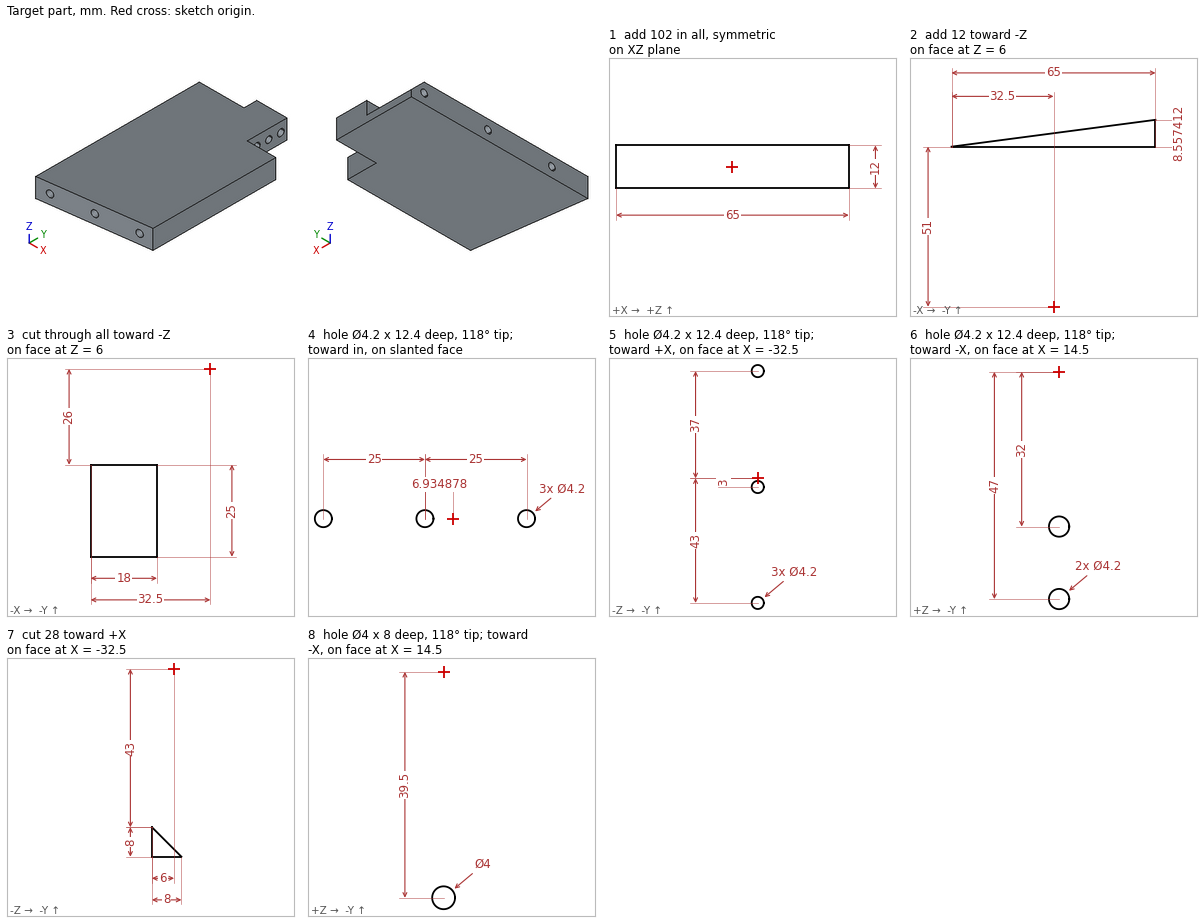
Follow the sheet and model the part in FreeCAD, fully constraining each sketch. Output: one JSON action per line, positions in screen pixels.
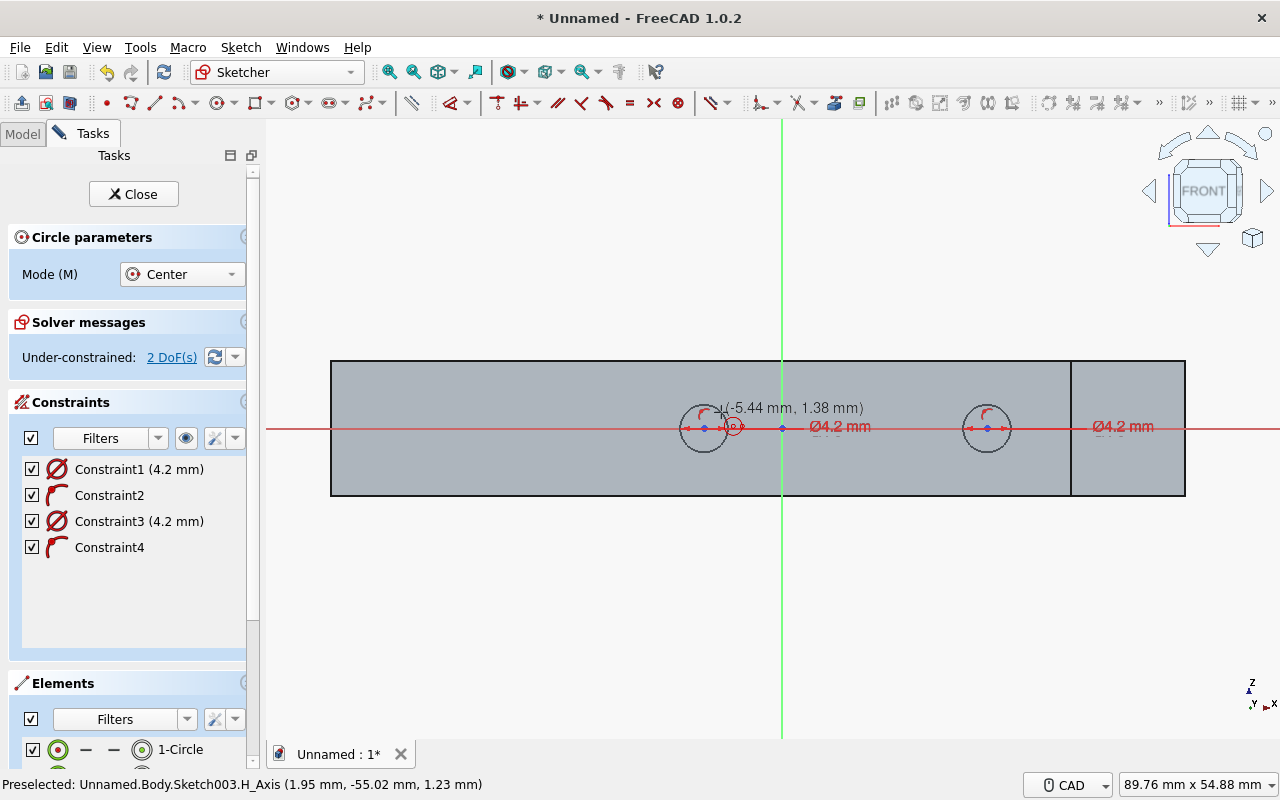
{"action": "left_click", "coordinate": [422, 429]}
{"action": "mouse_move", "coordinate": [438, 412]}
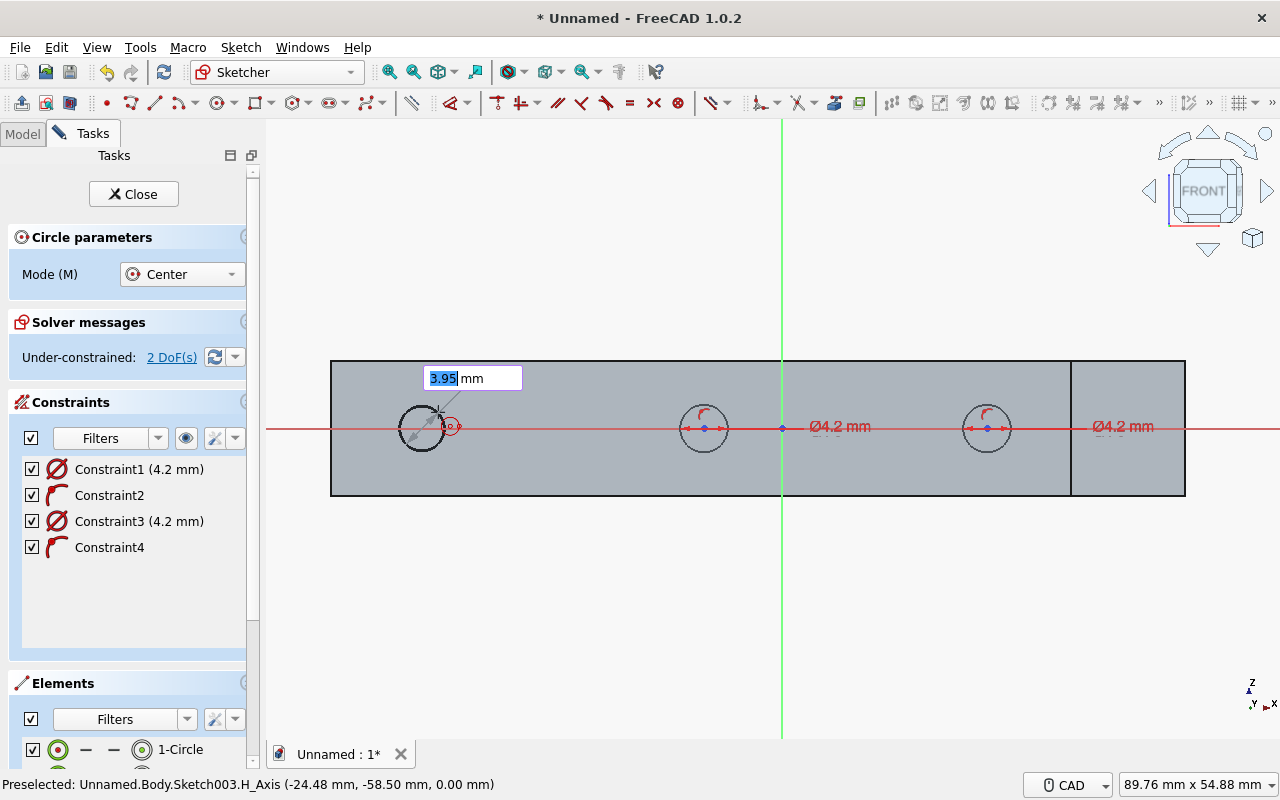
{"action": "type", "text": "4.2"}
{"action": "key", "text": "Return"}
{"action": "key", "text": "Escape"}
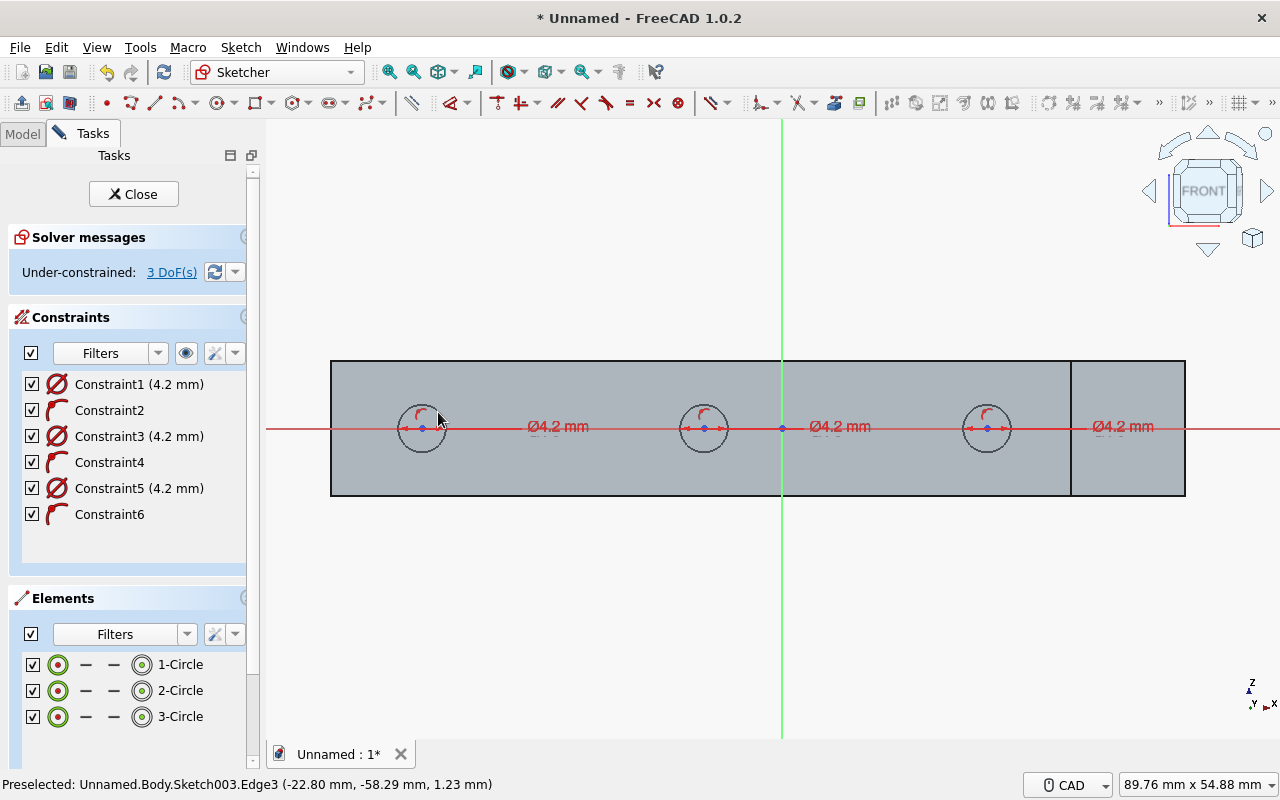
{"action": "key", "text": "d"}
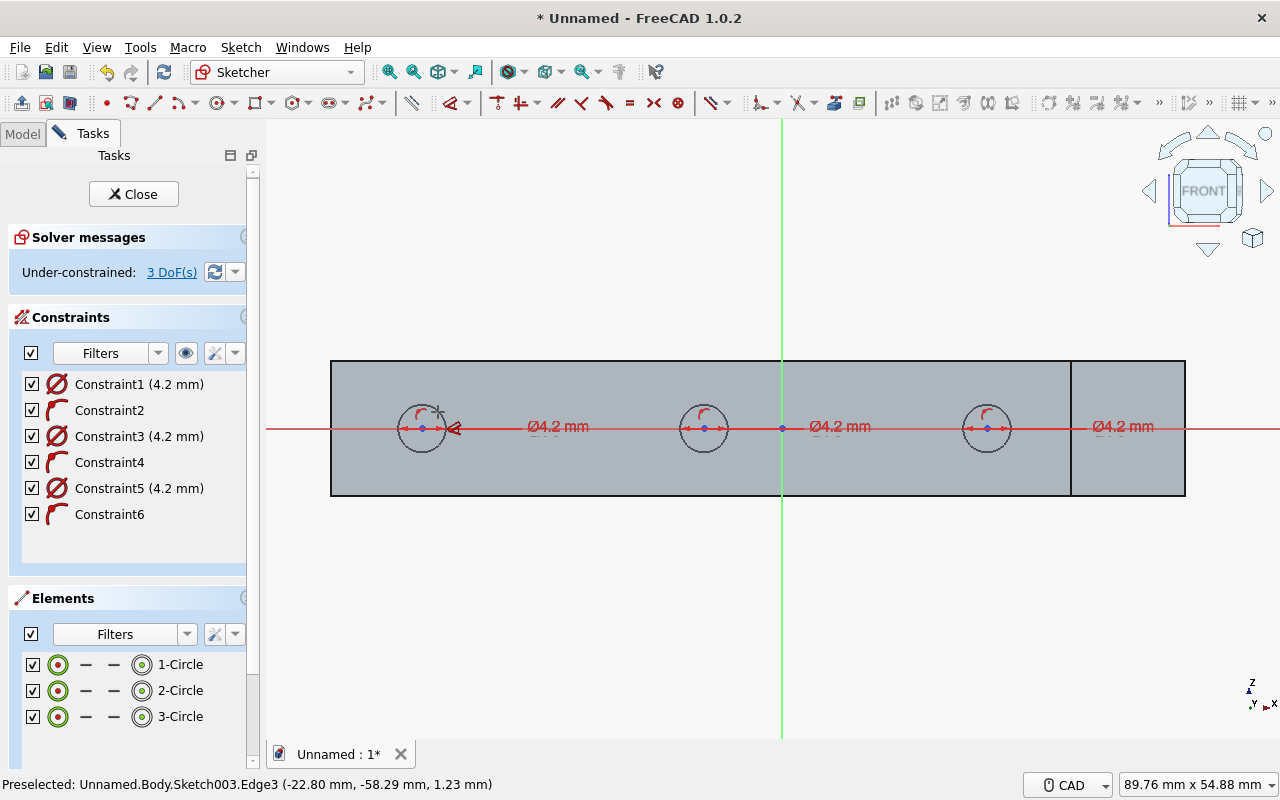
{"action": "left_click", "coordinate": [987, 429]}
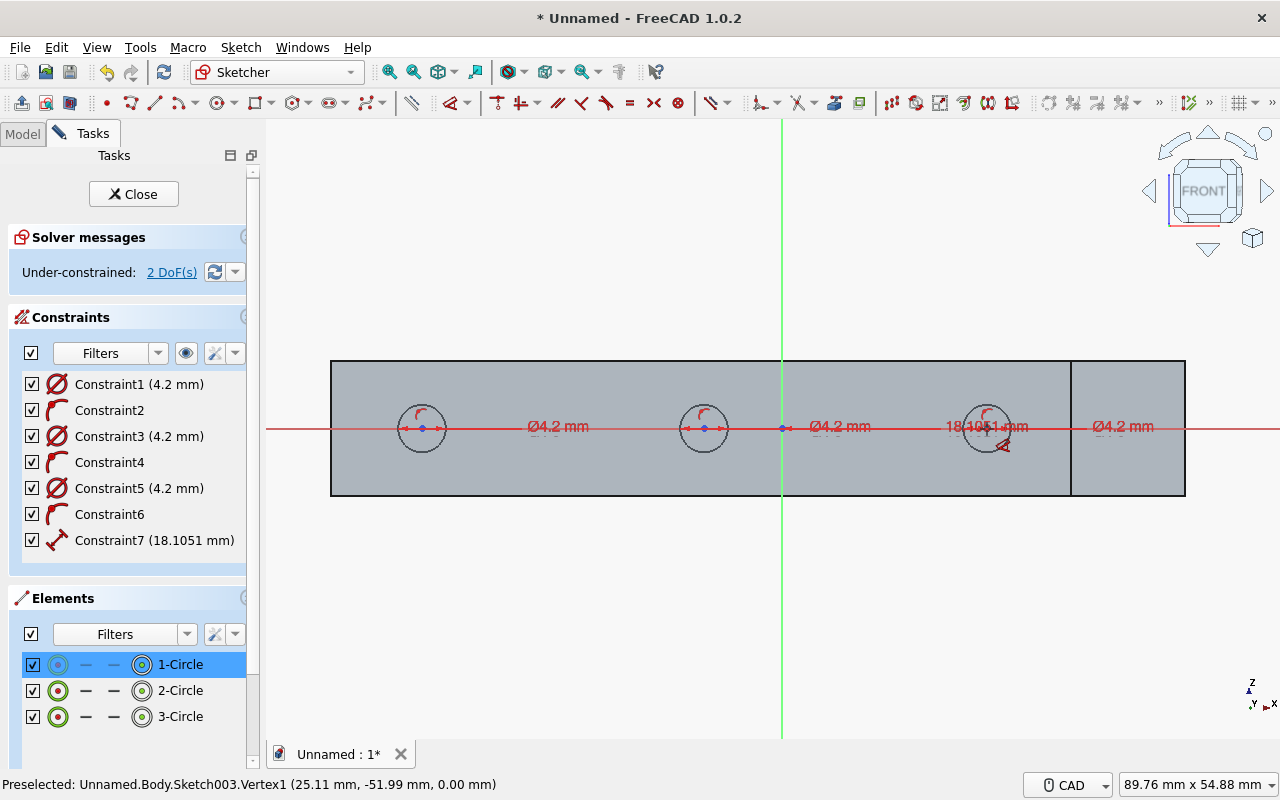
{"action": "left_click", "coordinate": [704, 429]}
{"action": "left_click", "coordinate": [845, 463]}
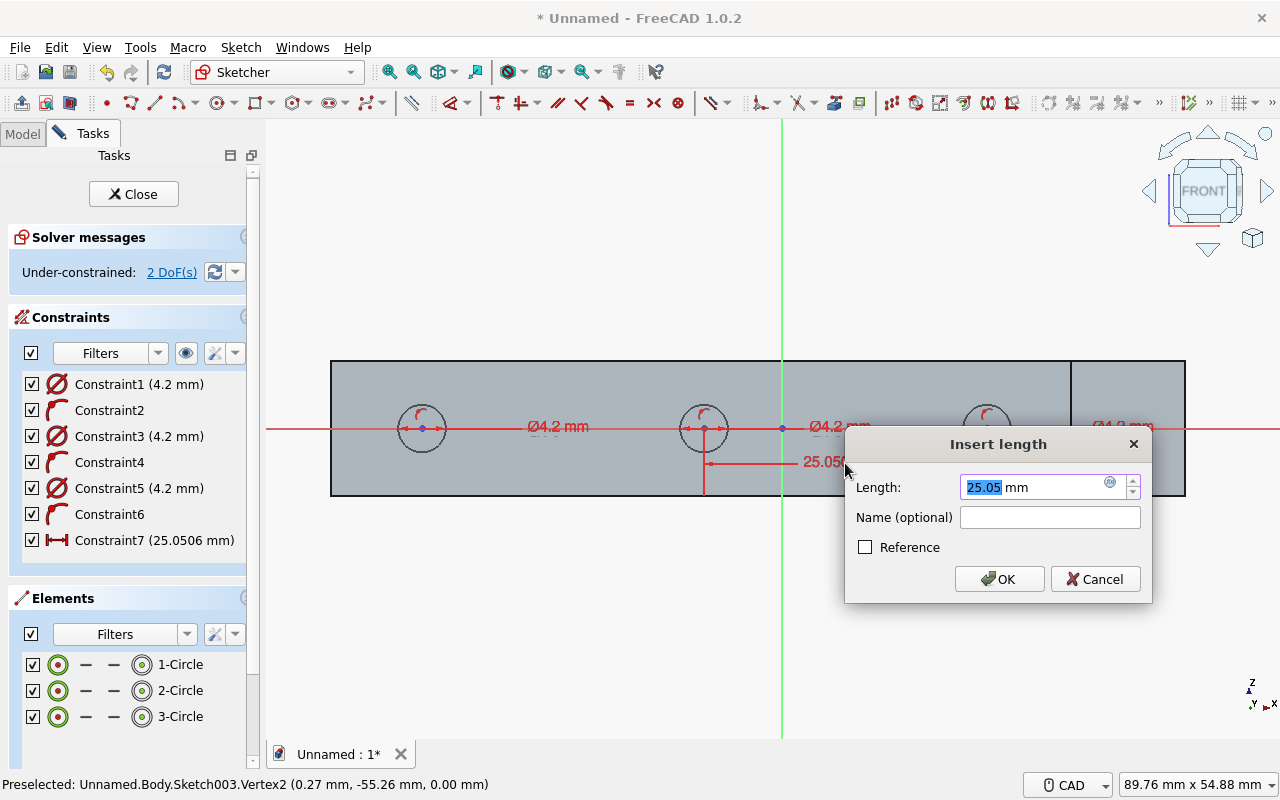
{"action": "type", "text": "25"}
{"action": "key", "text": "Return"}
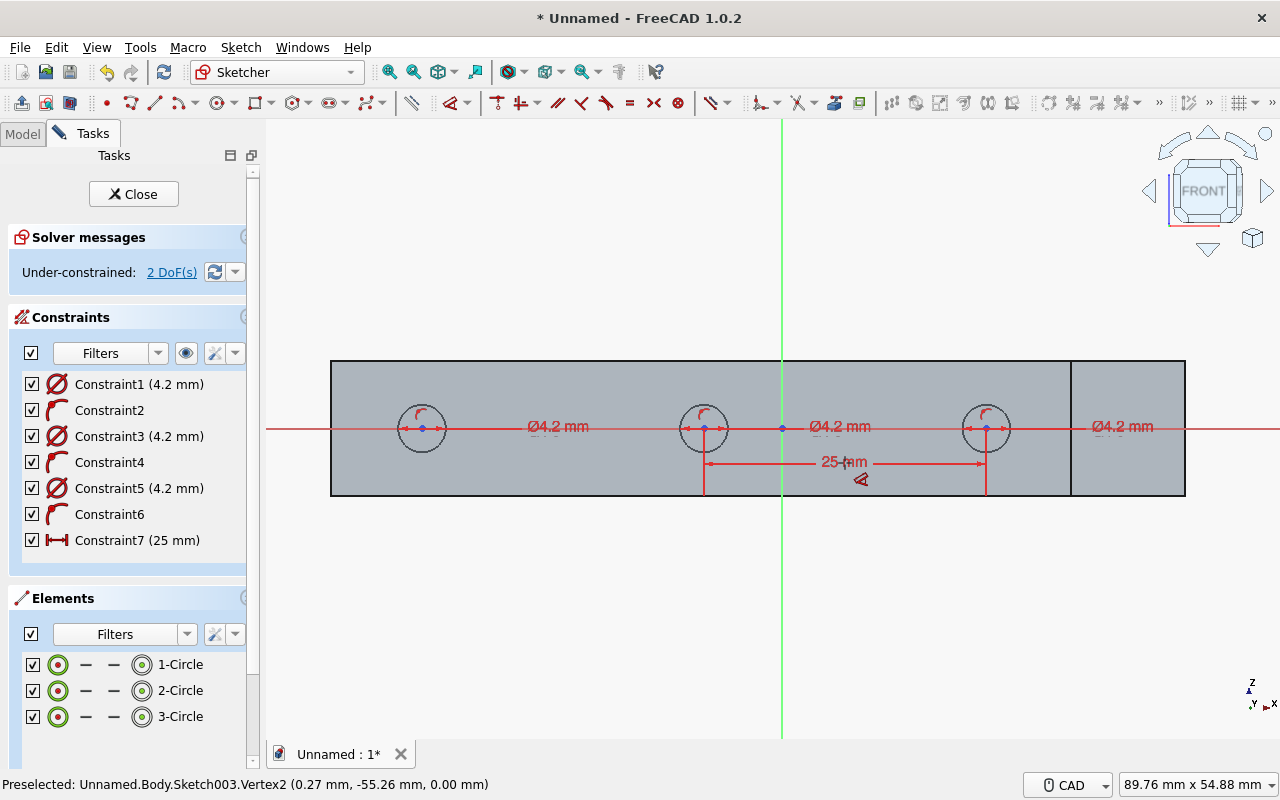
{"action": "left_click", "coordinate": [704, 429]}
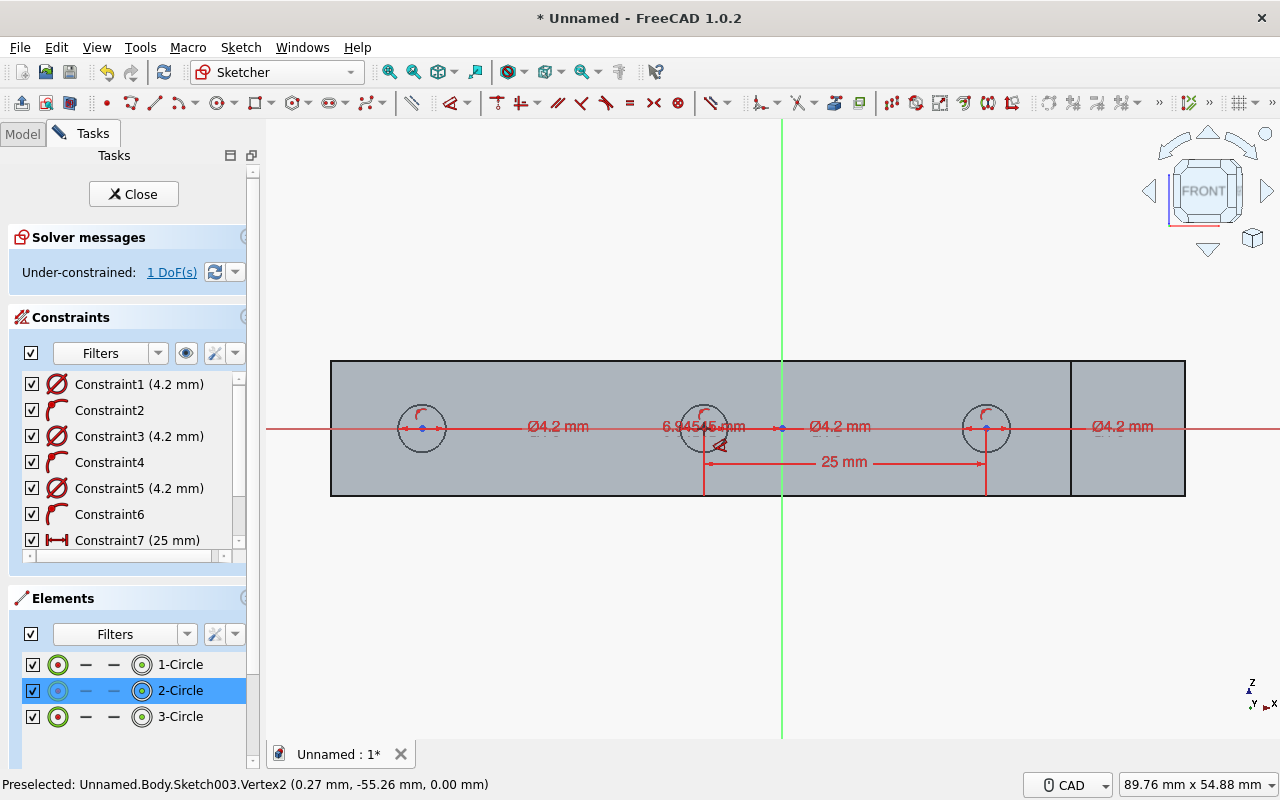
{"action": "left_click", "coordinate": [422, 429]}
{"action": "left_click", "coordinate": [563, 463]}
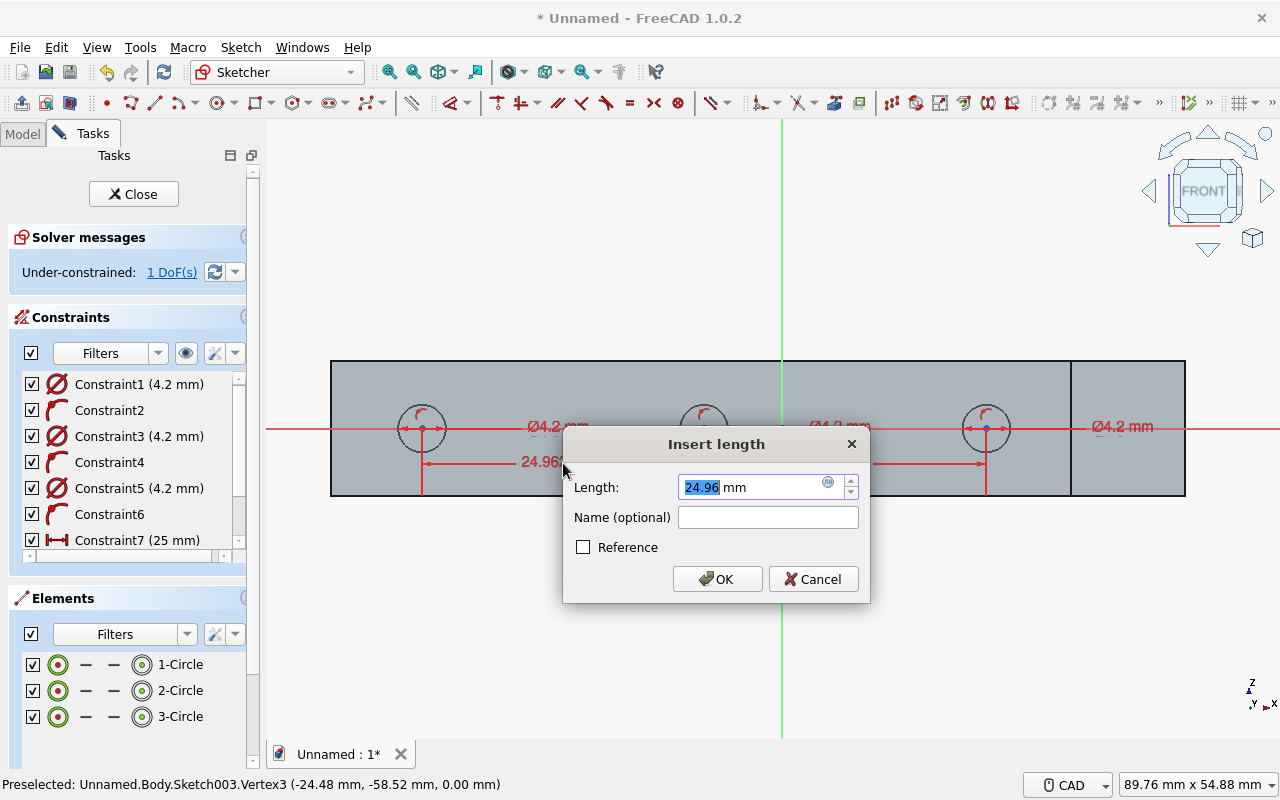
{"action": "type", "text": "25"}
{"action": "key", "text": "Return"}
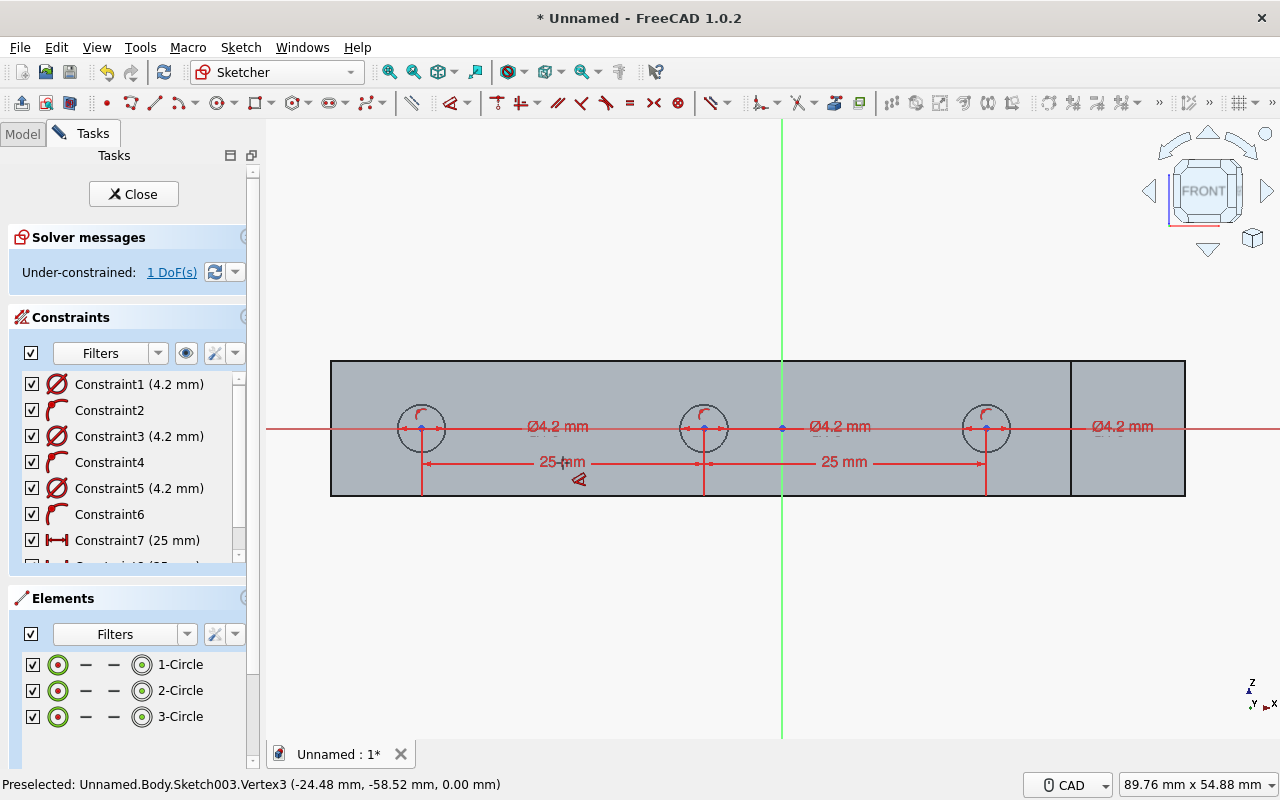
{"action": "left_click", "coordinate": [704, 429]}
{"action": "left_click", "coordinate": [743, 463]}